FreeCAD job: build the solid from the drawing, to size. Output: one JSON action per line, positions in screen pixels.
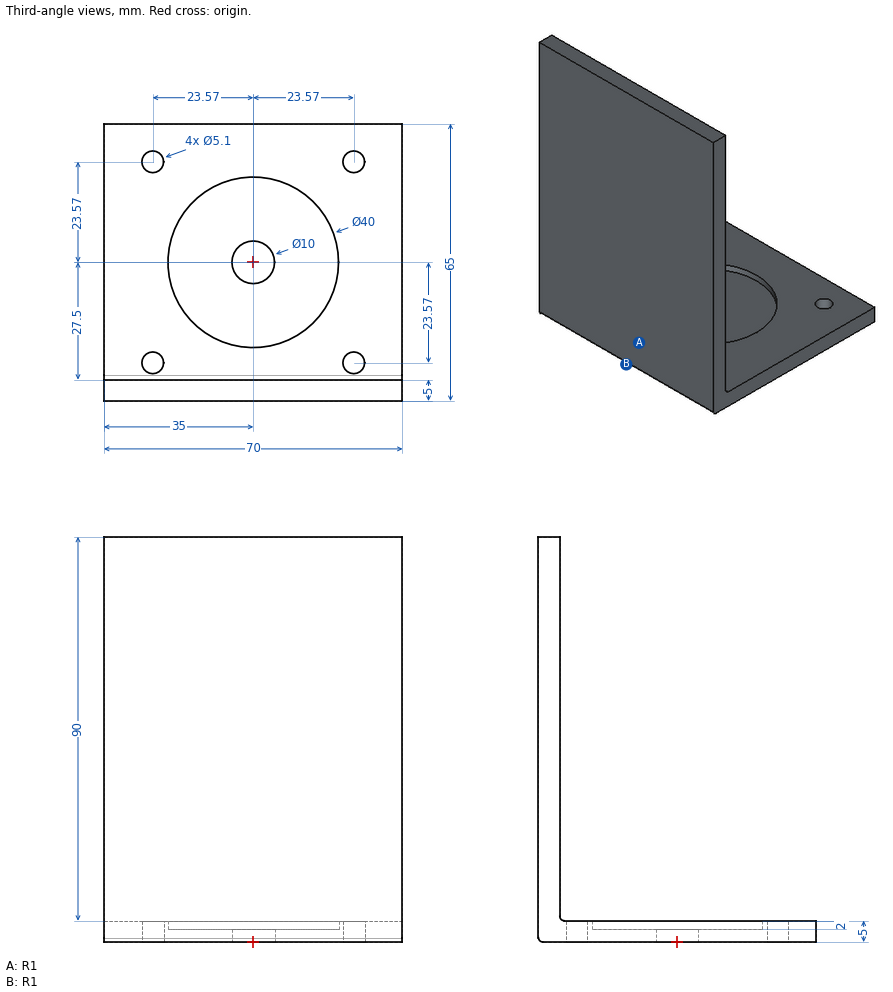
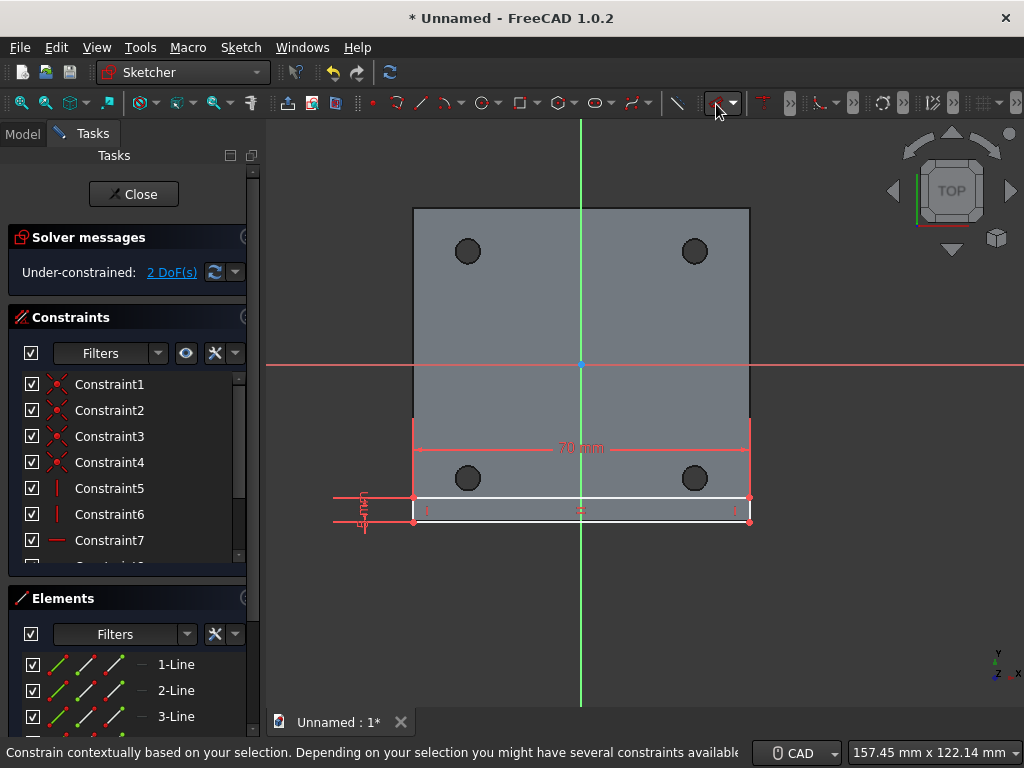
{"action": "left_click", "coordinate": [413, 498]}
{"action": "left_click", "coordinate": [497, 331]}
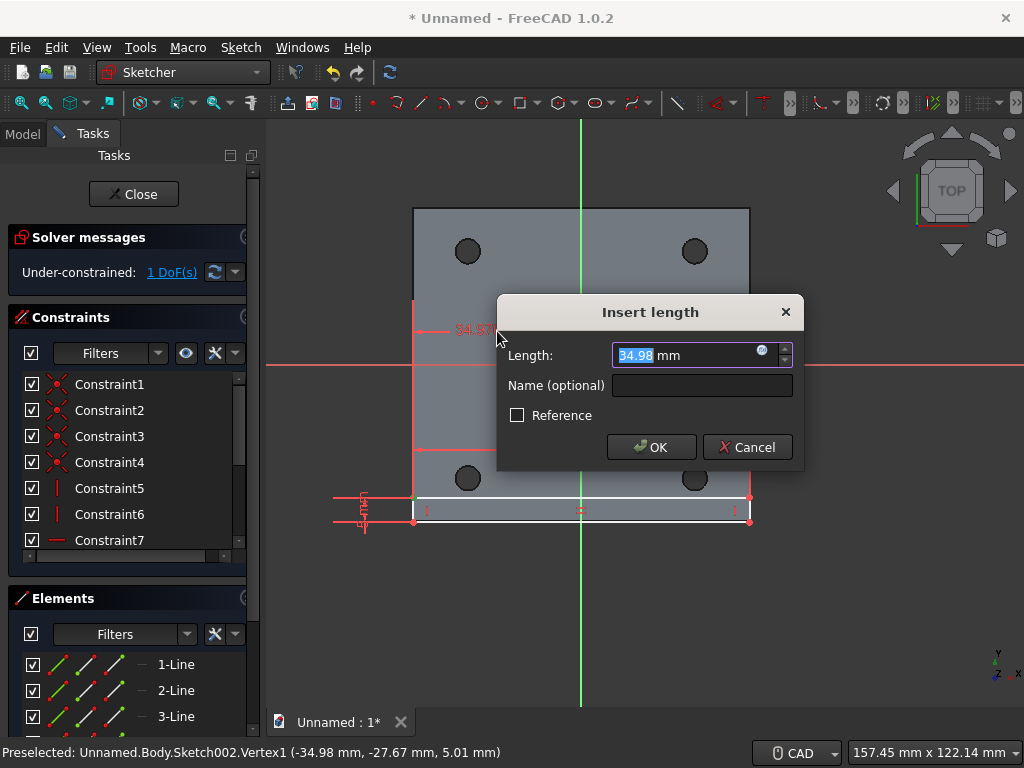
{"action": "type", "text": "35"}
{"action": "key", "text": "Return"}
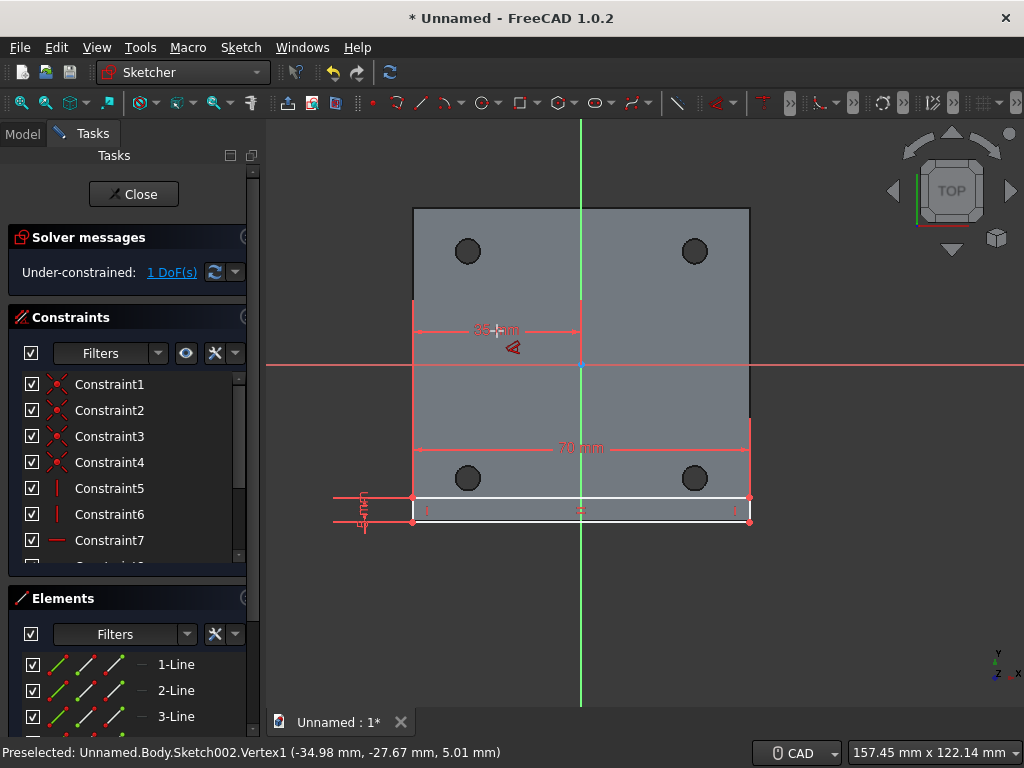
{"action": "left_click", "coordinate": [413, 498]}
{"action": "left_click", "coordinate": [379, 431]}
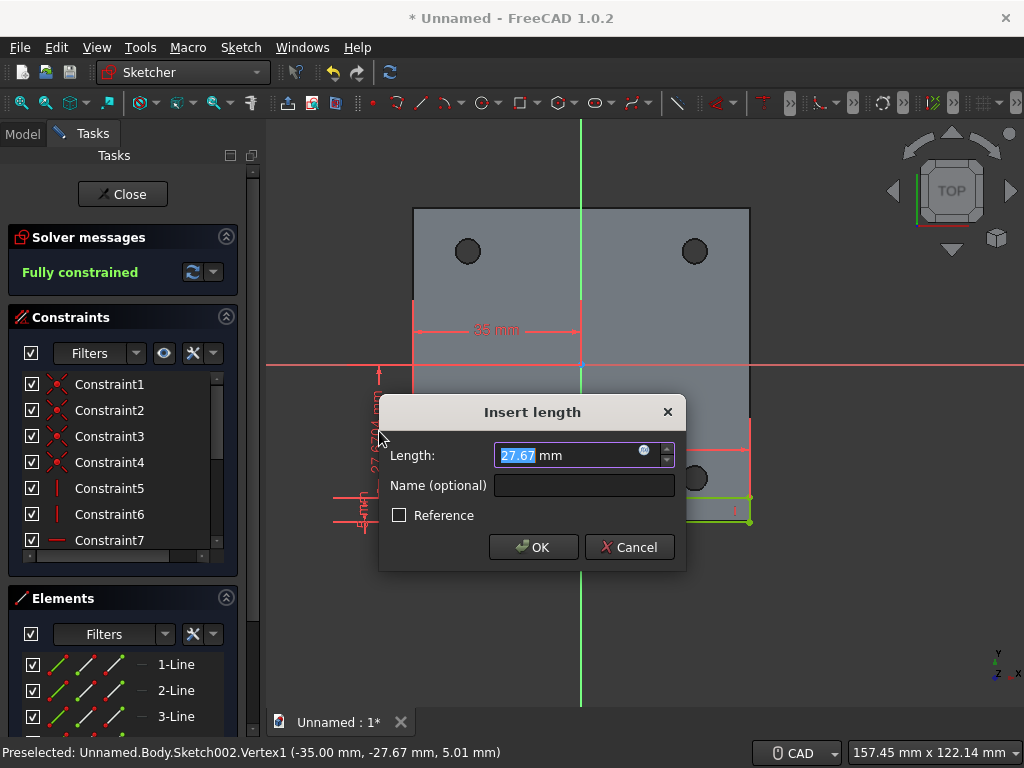
{"action": "type", "text": "27.5"}
{"action": "key", "text": "Return"}
{"action": "key", "text": "Escape"}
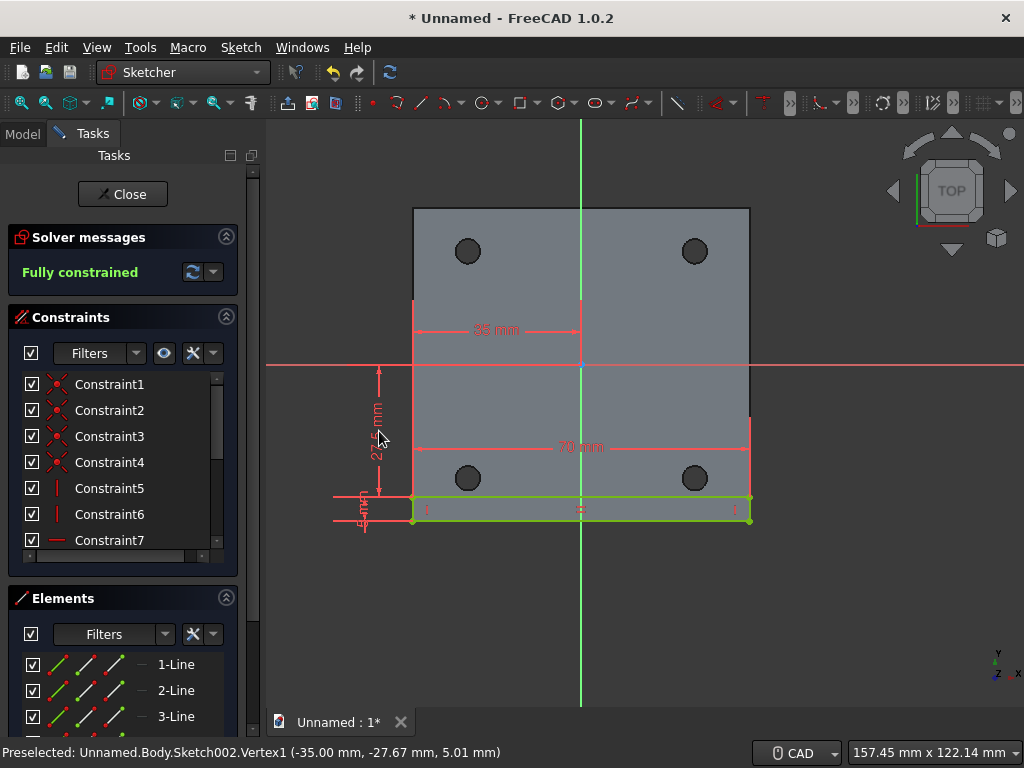
{"action": "left_click", "coordinate": [123, 194]}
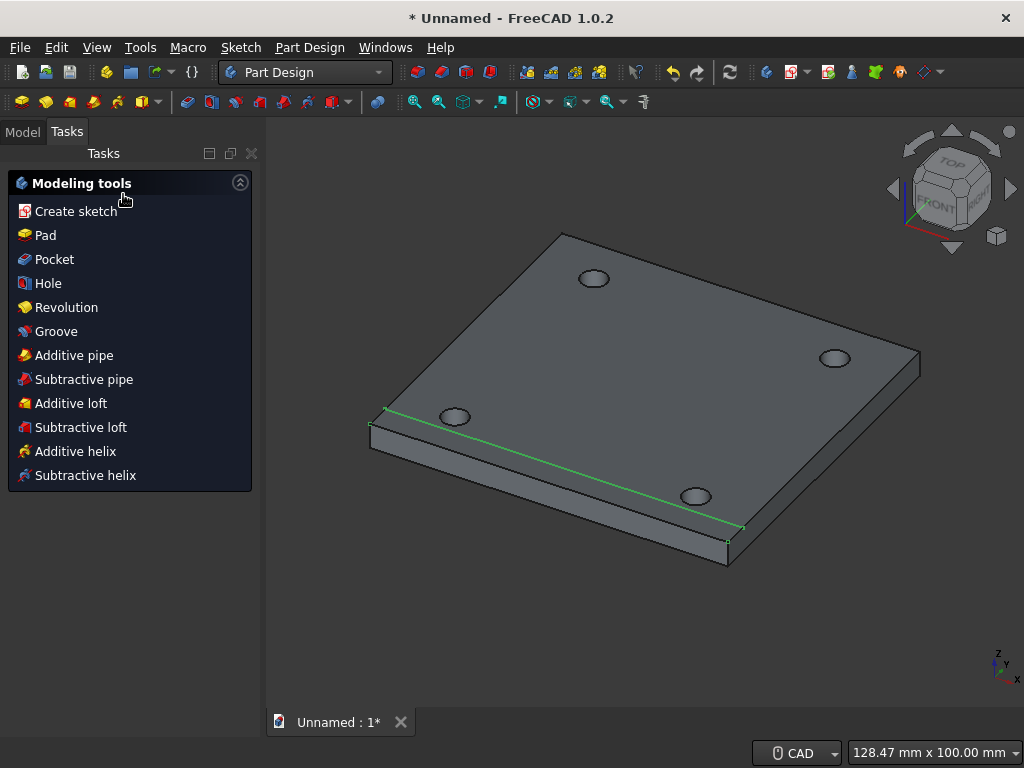
{"action": "left_click", "coordinate": [22, 102]}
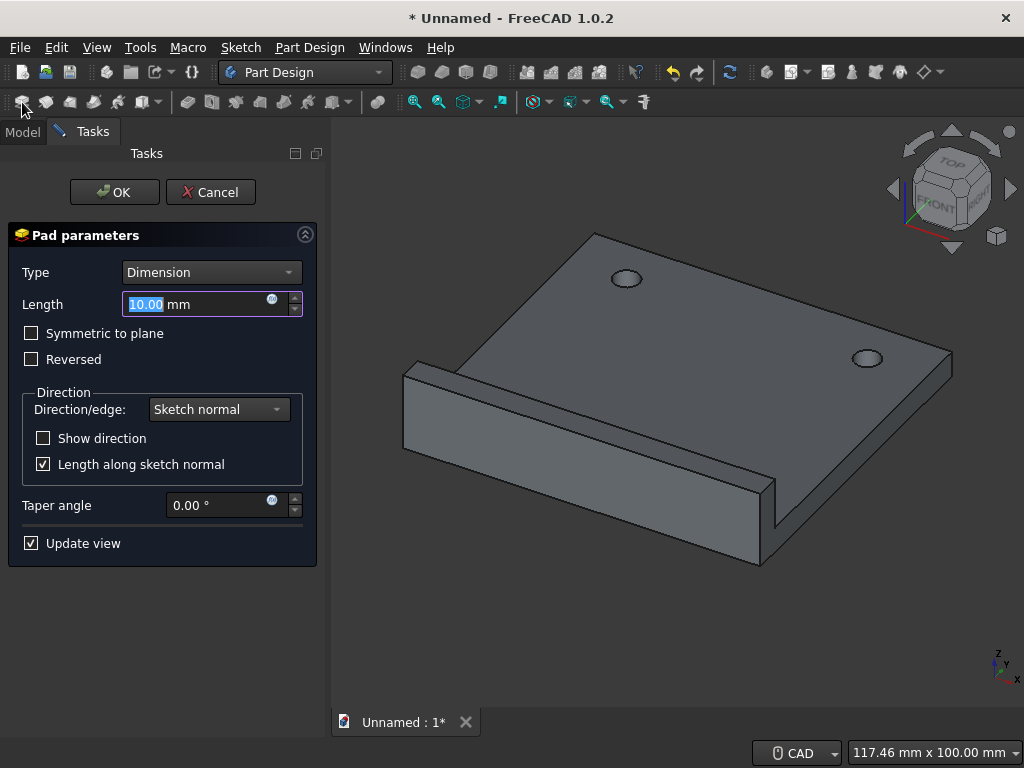
{"action": "type", "text": "90"}
{"action": "key", "text": "Tab"}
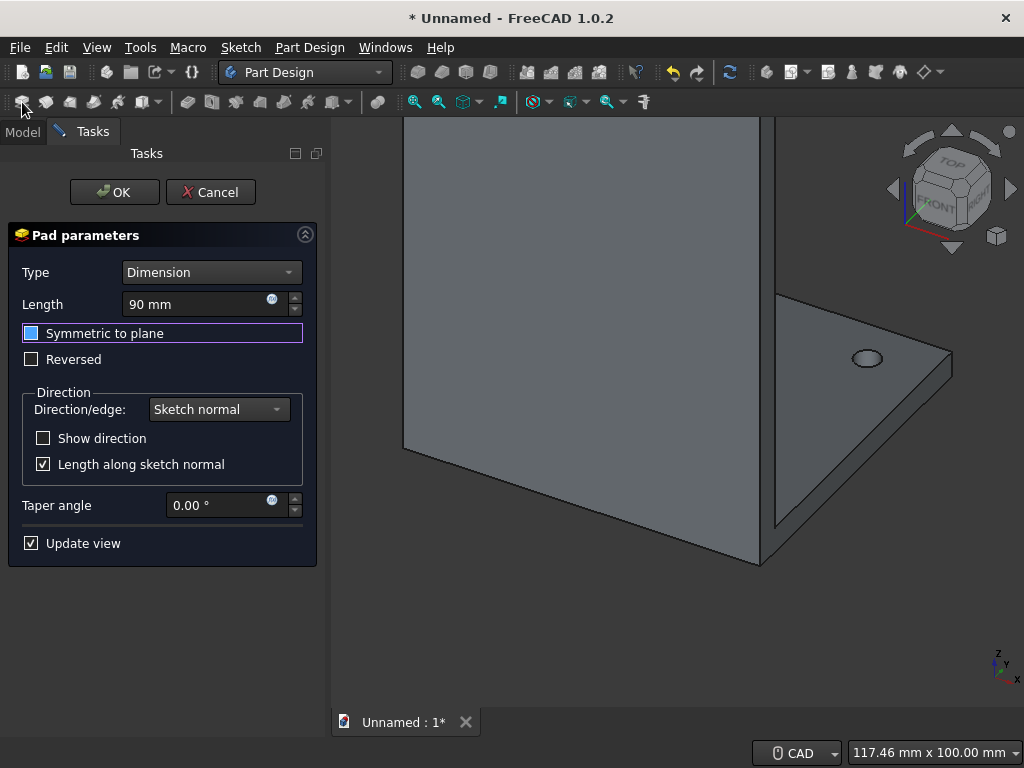
{"action": "left_click", "coordinate": [115, 192]}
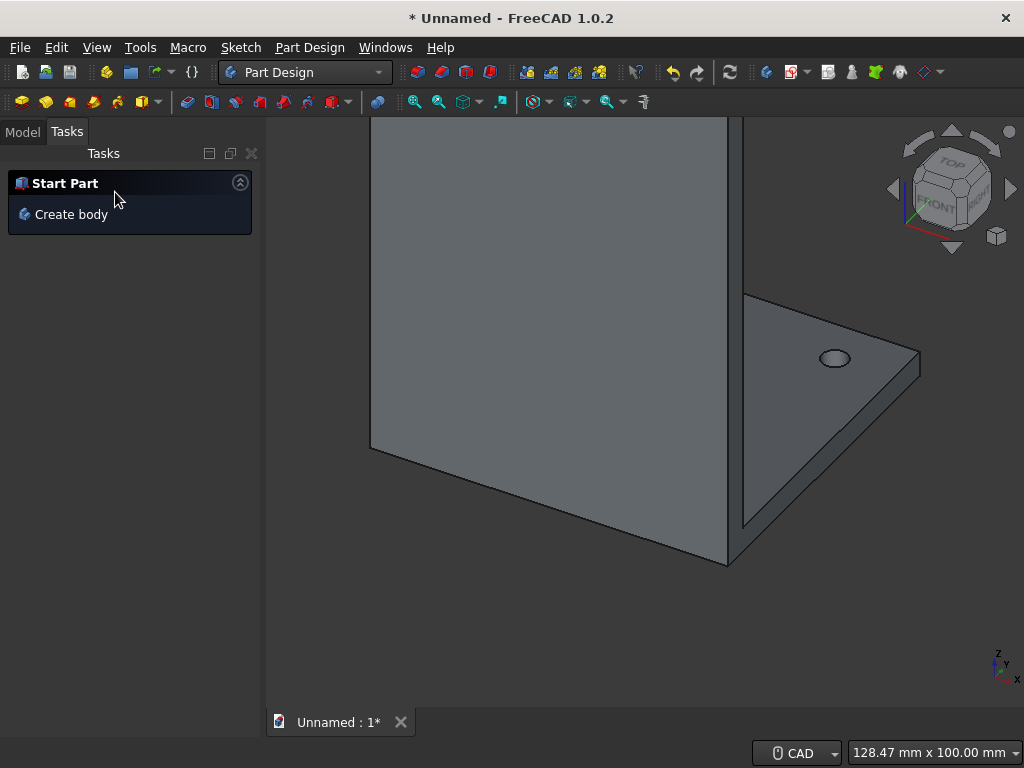
{"action": "left_click", "coordinate": [416, 102]}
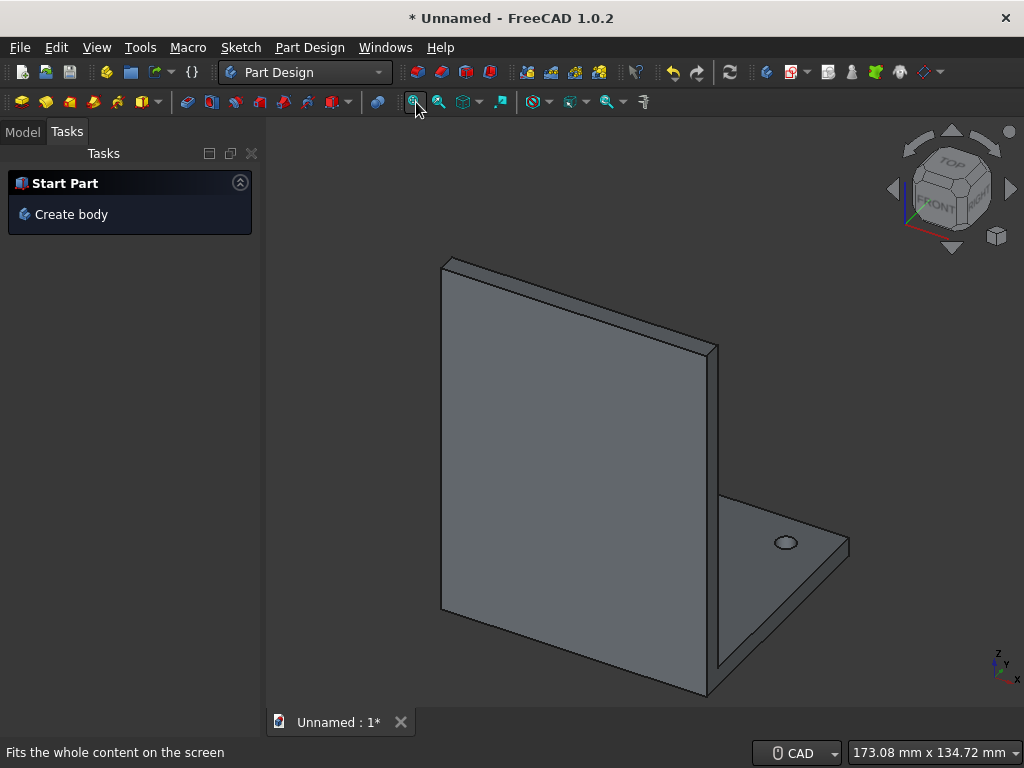
{"action": "key", "text": "0"}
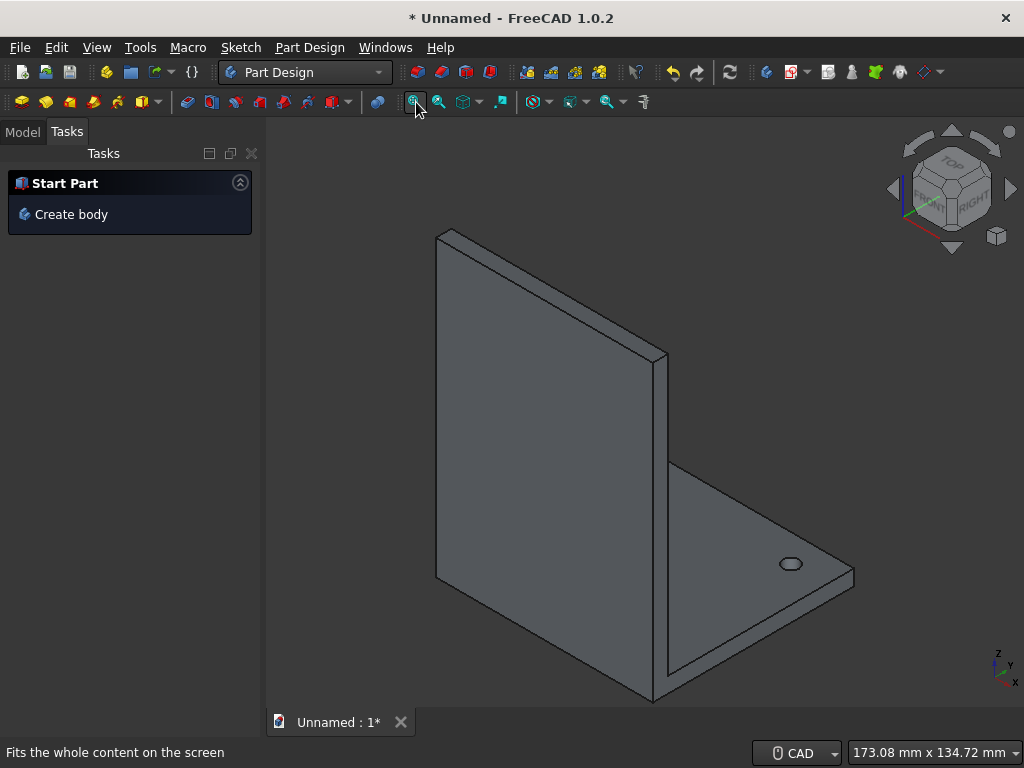
{"action": "key", "text": "2"}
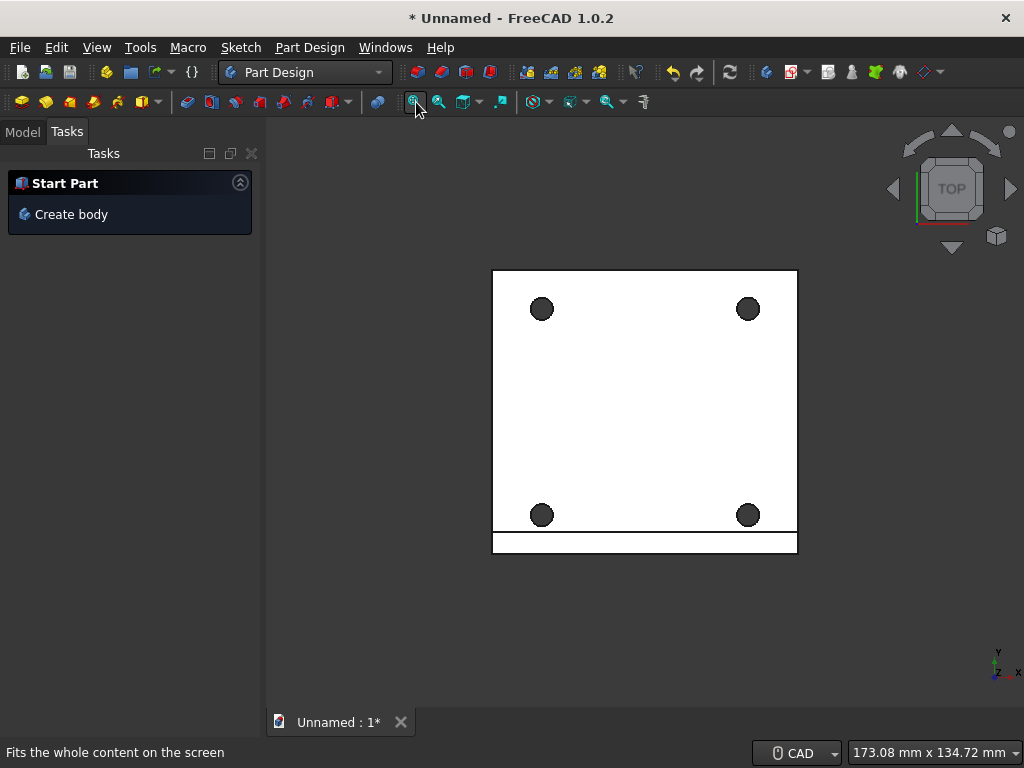
{"action": "key", "text": "1"}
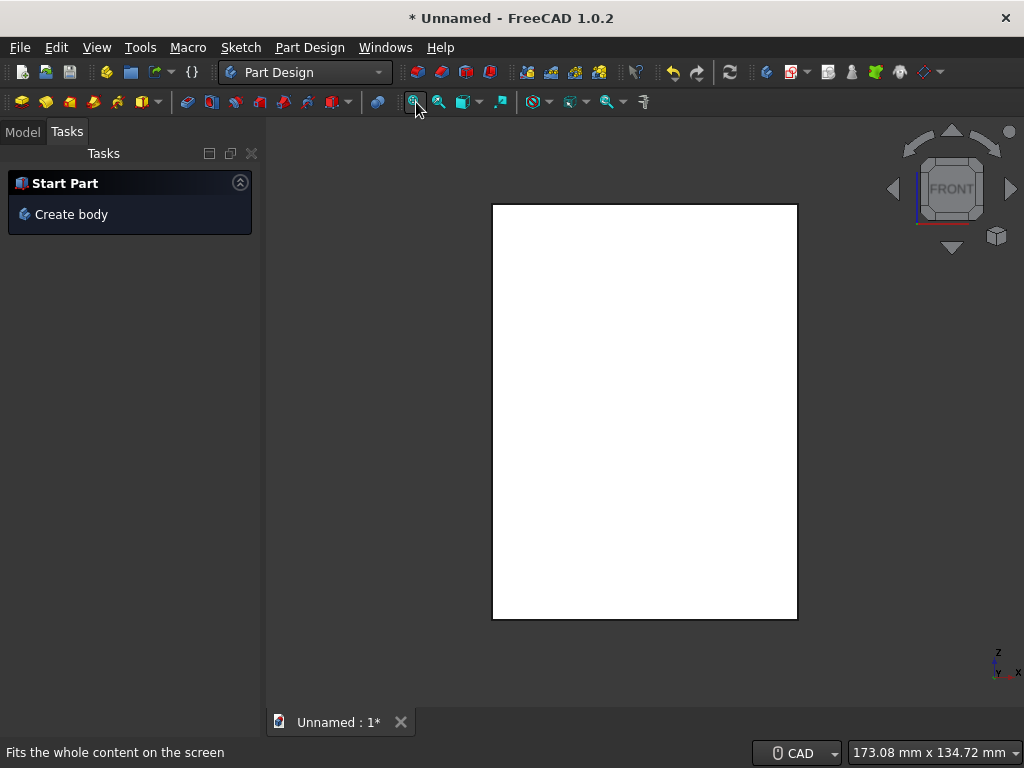
{"action": "key", "text": "3"}